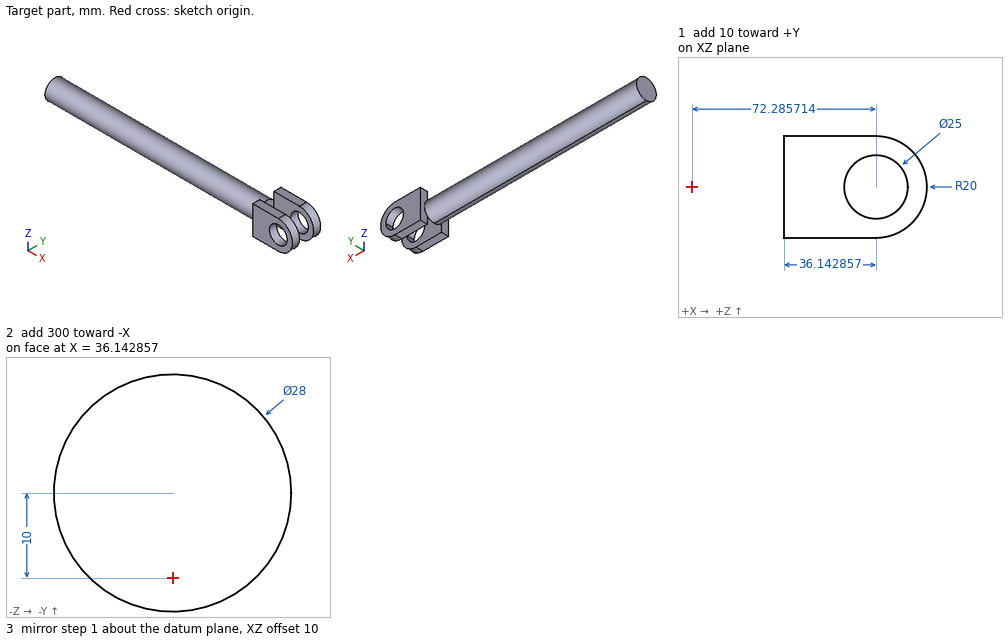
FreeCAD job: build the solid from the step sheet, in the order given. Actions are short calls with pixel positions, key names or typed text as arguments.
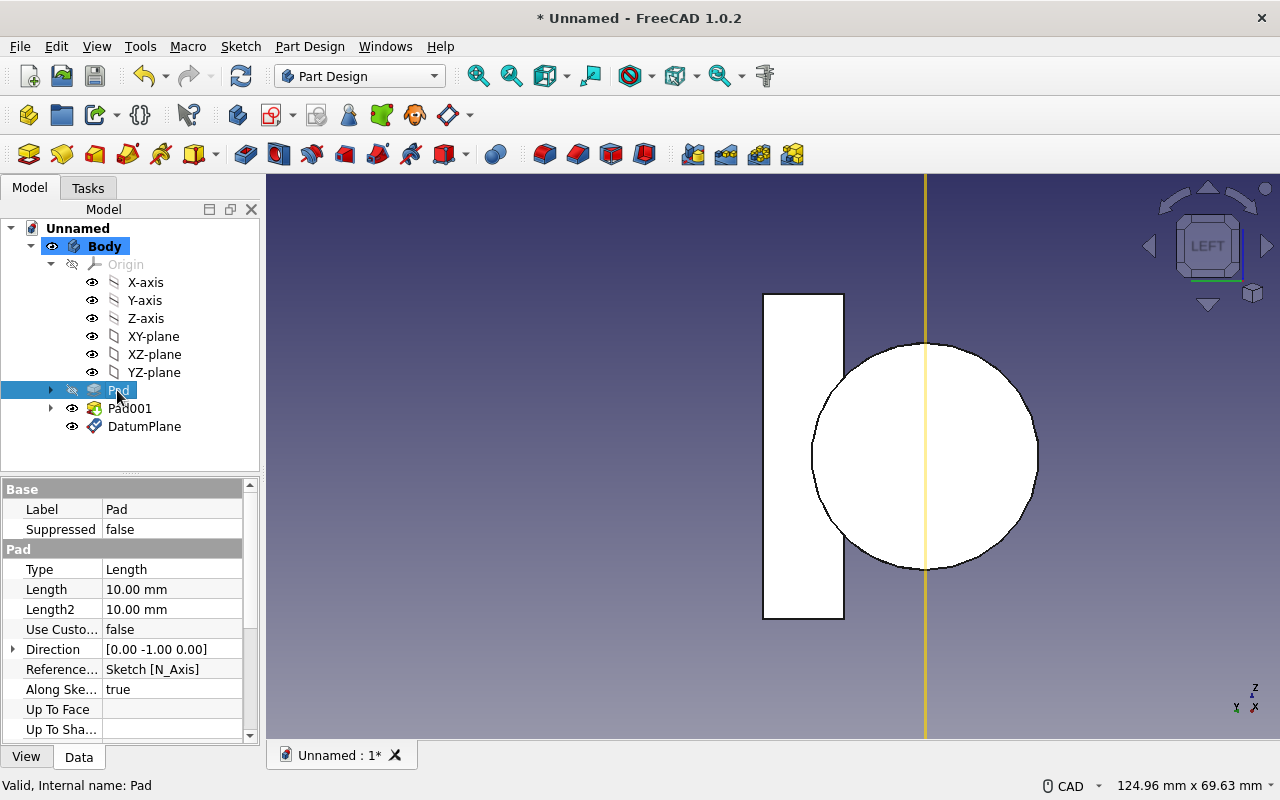
click(693, 154)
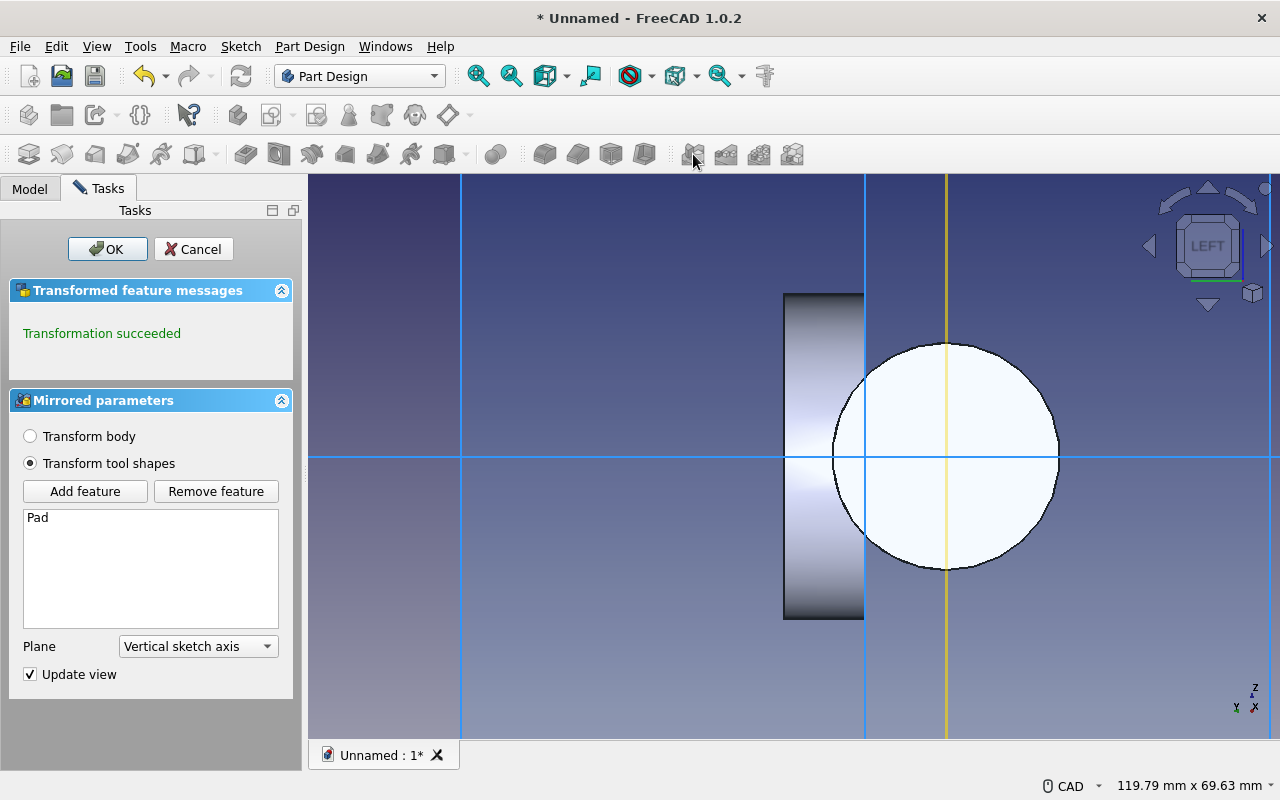
click(199, 646)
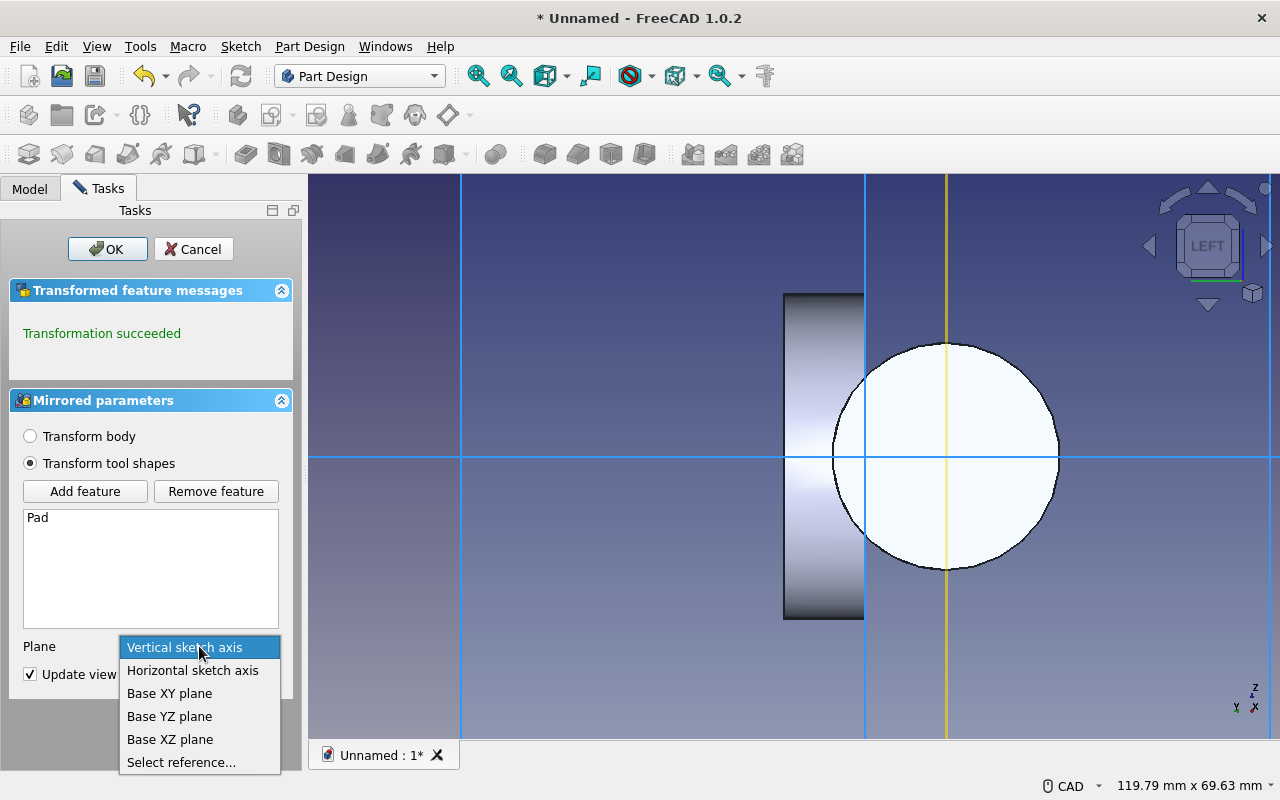
click(198, 762)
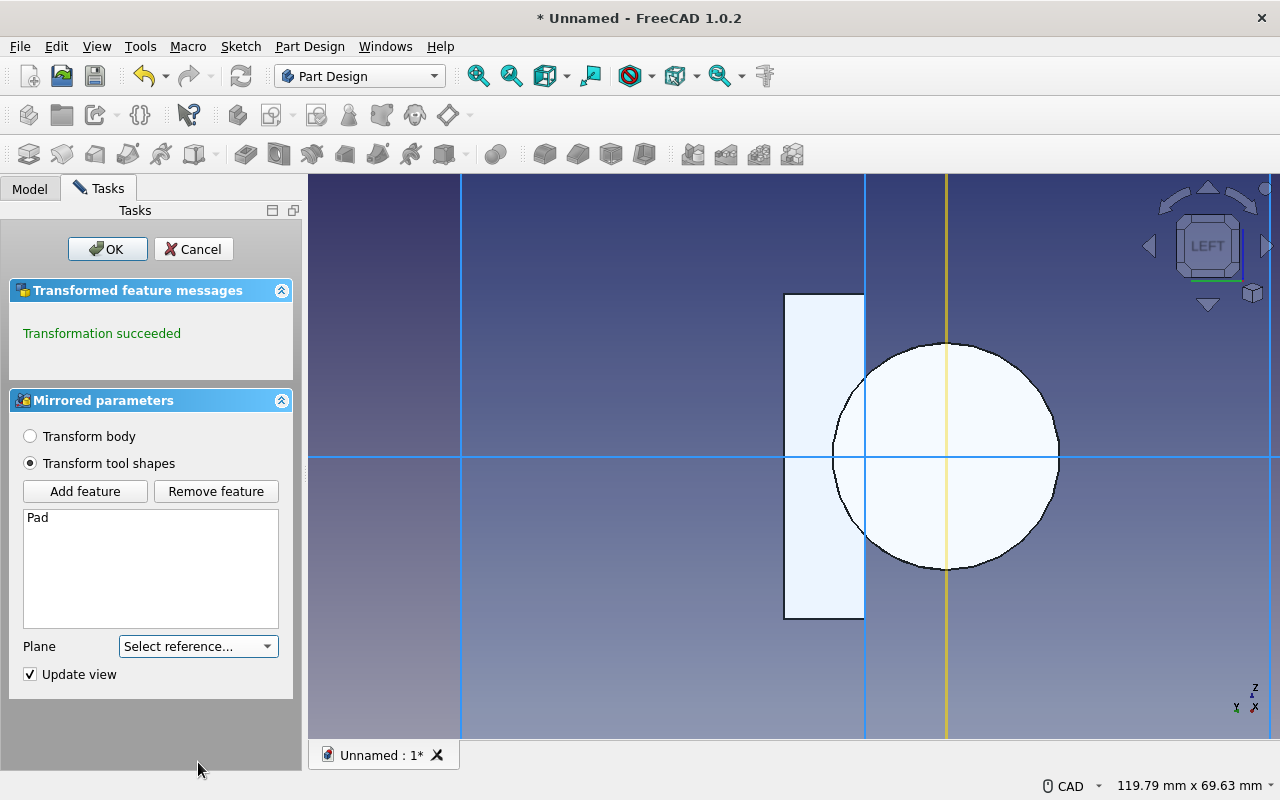
click(30, 188)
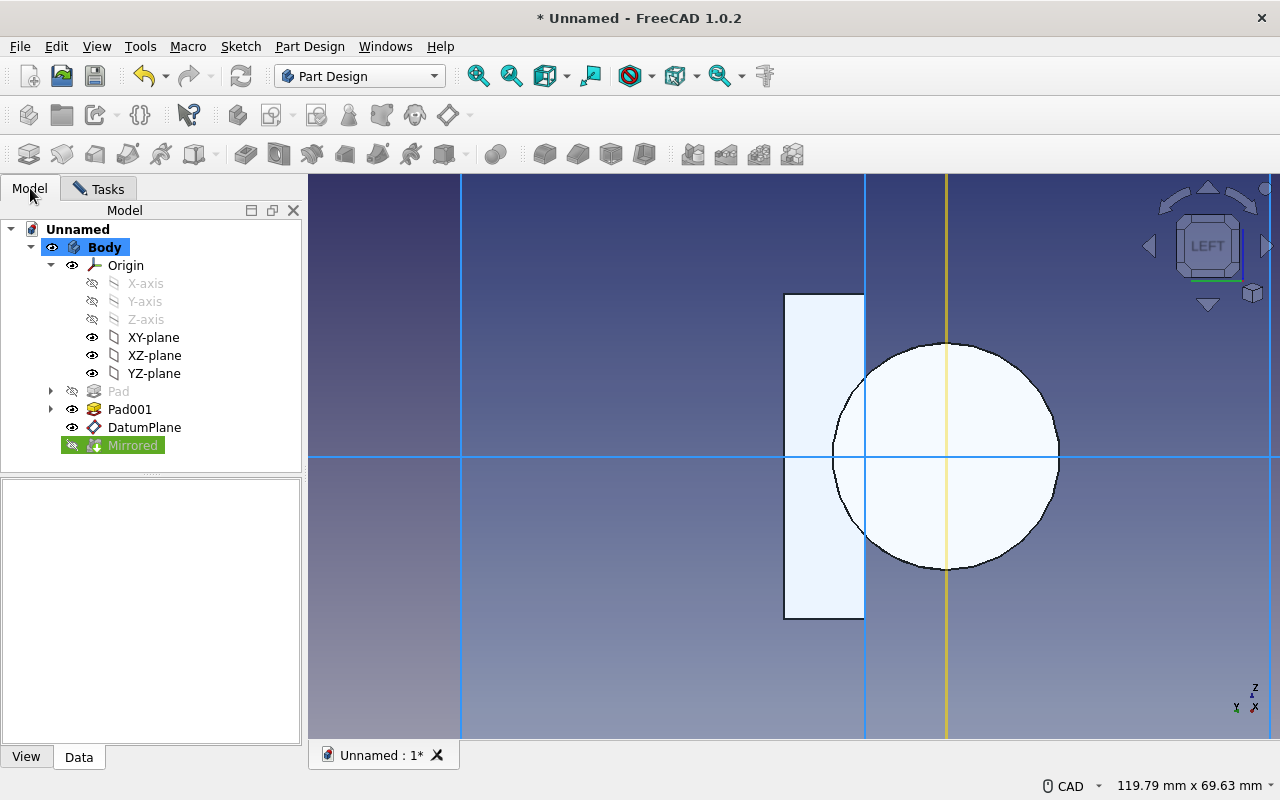
click(117, 427)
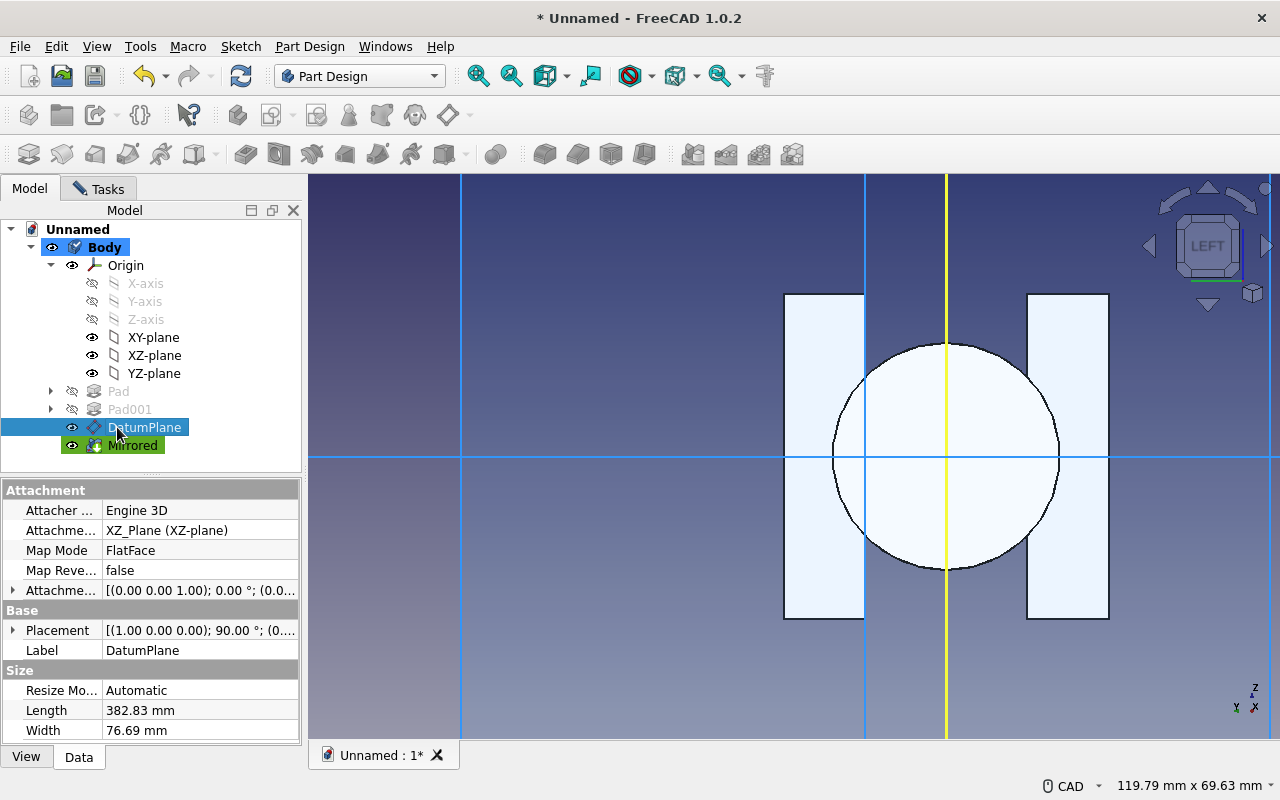
click(98, 188)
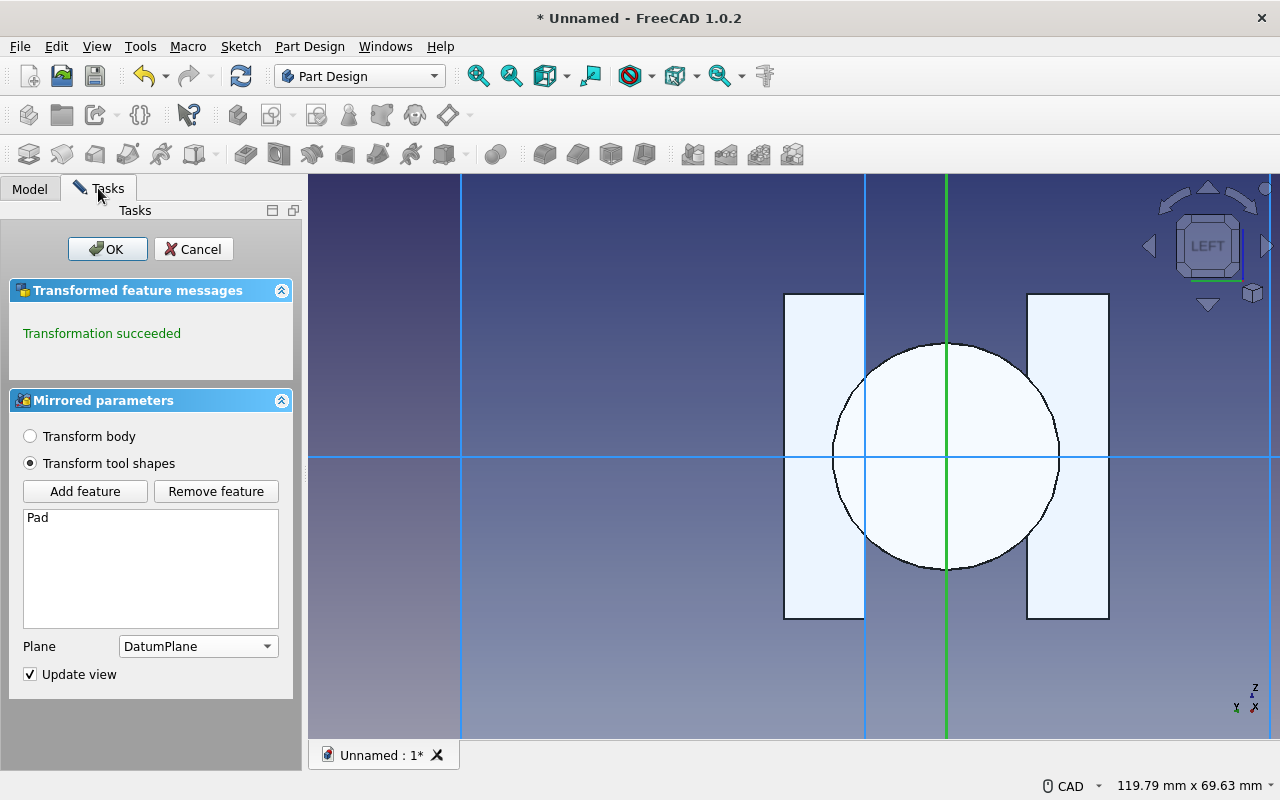
click(108, 249)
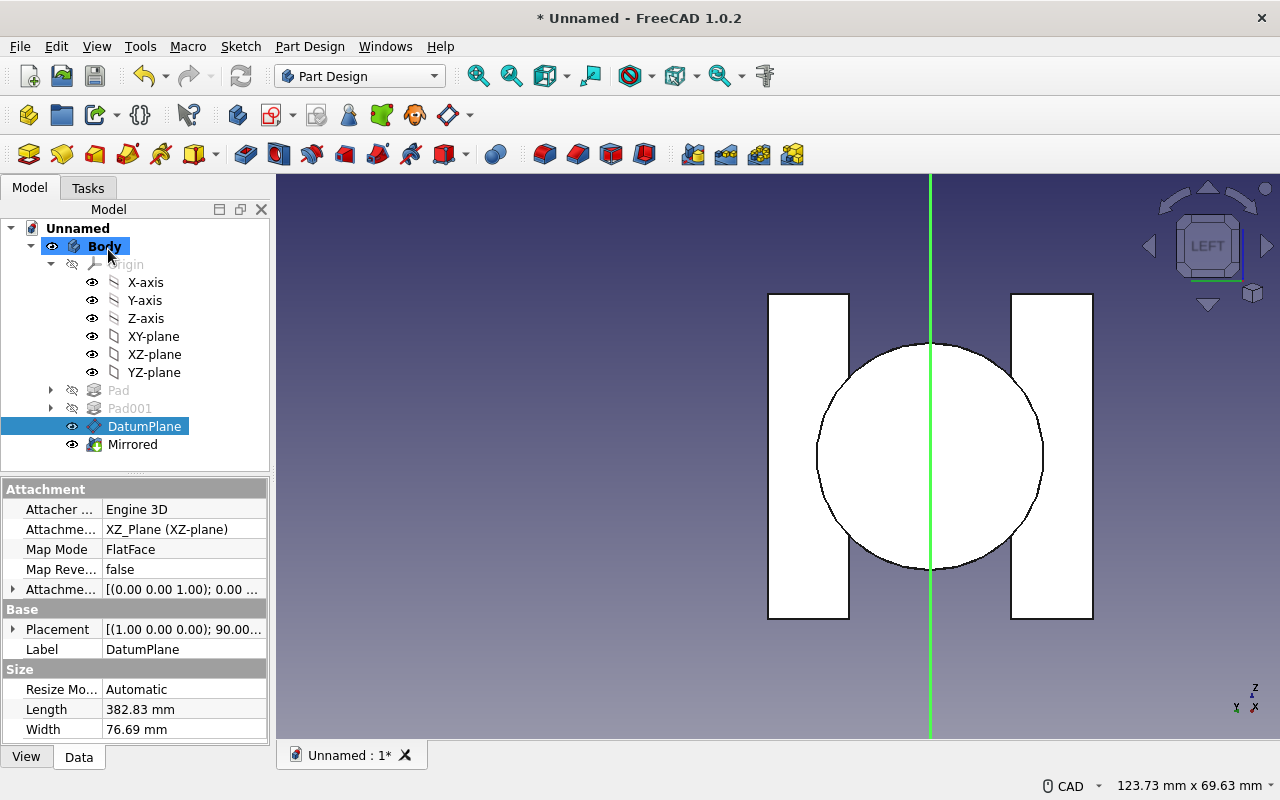
click(117, 426)
key(space)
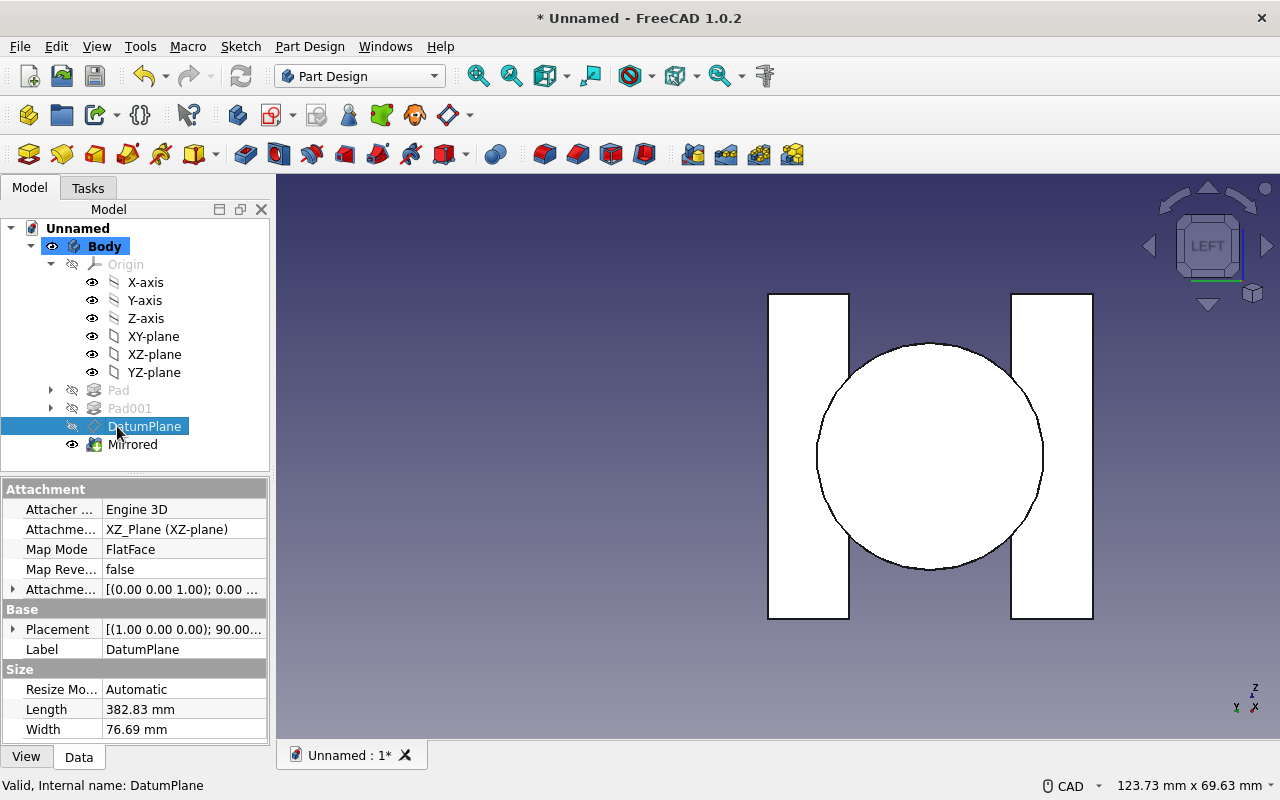
key(0)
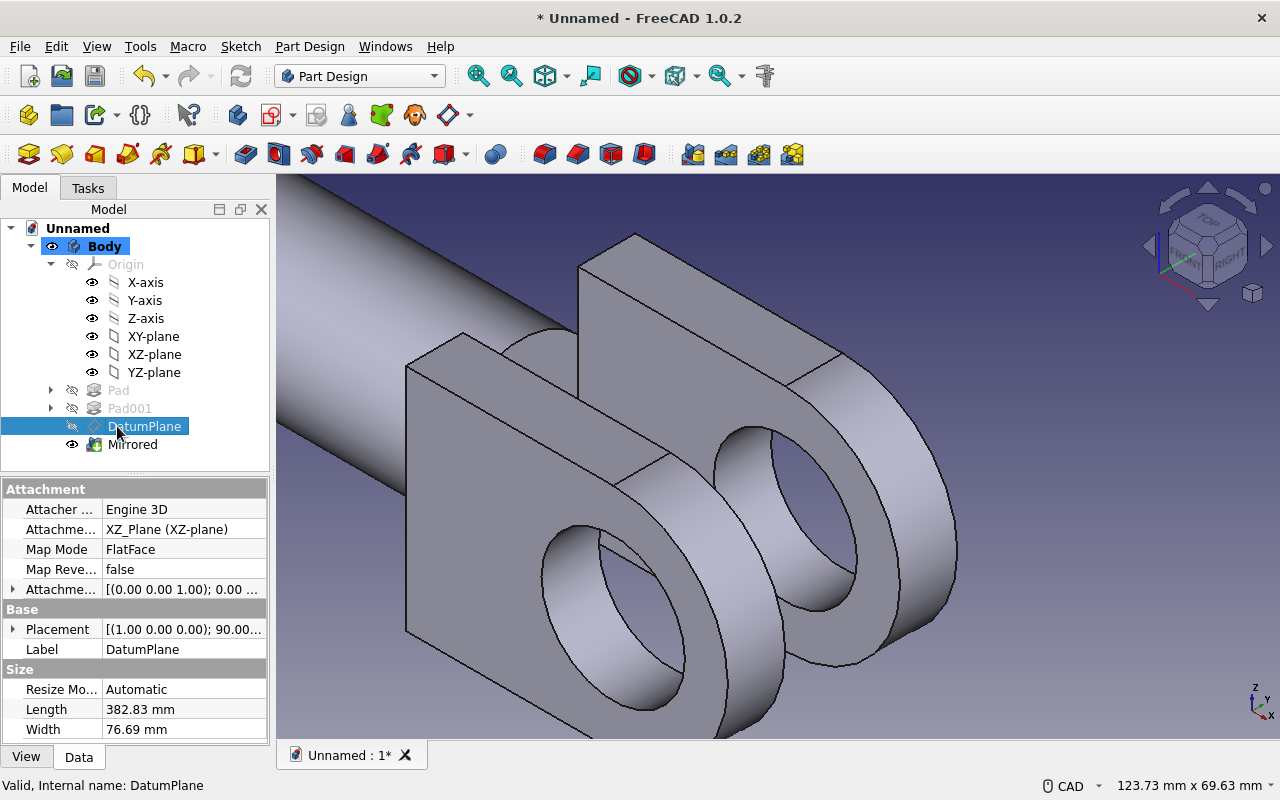
key(v)
key(f)